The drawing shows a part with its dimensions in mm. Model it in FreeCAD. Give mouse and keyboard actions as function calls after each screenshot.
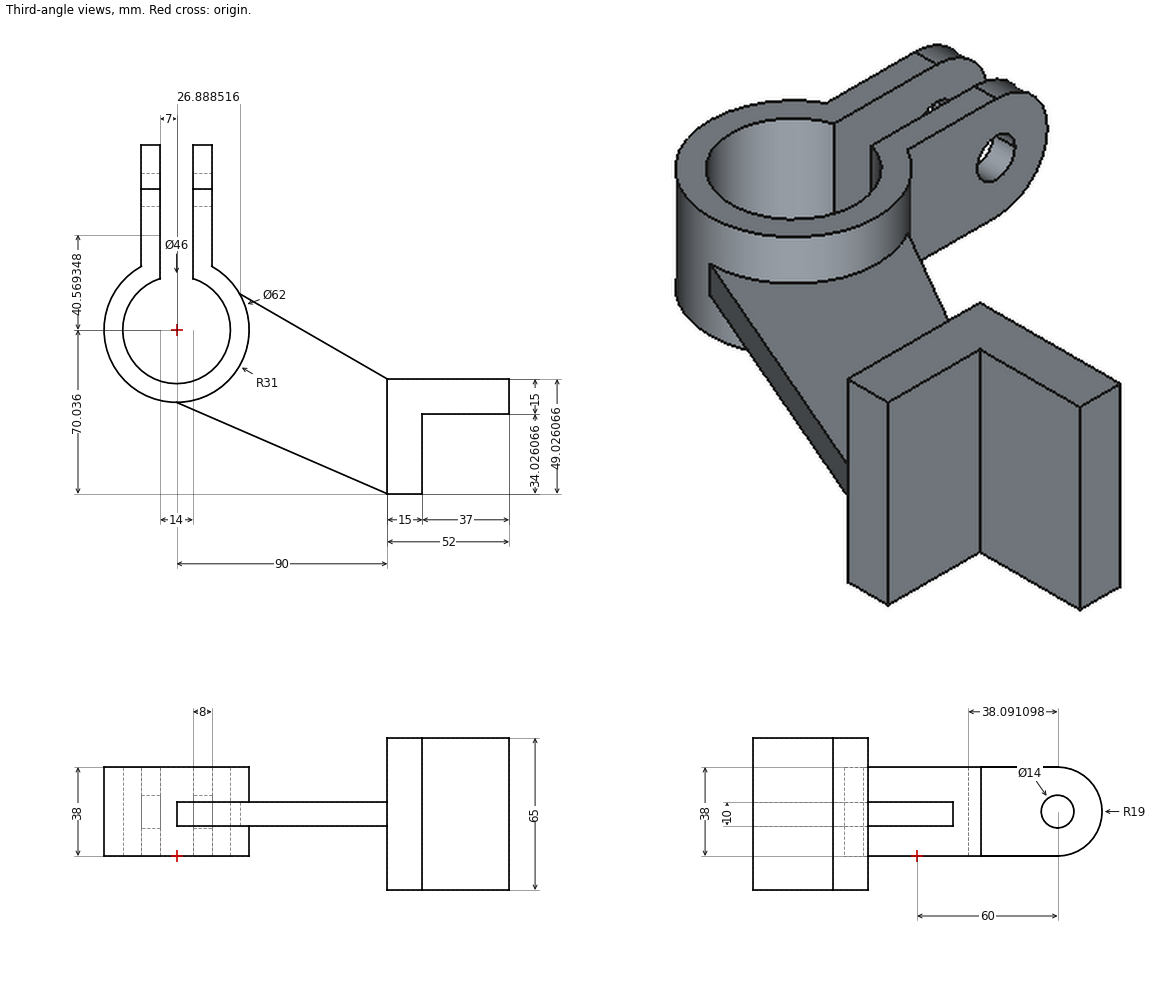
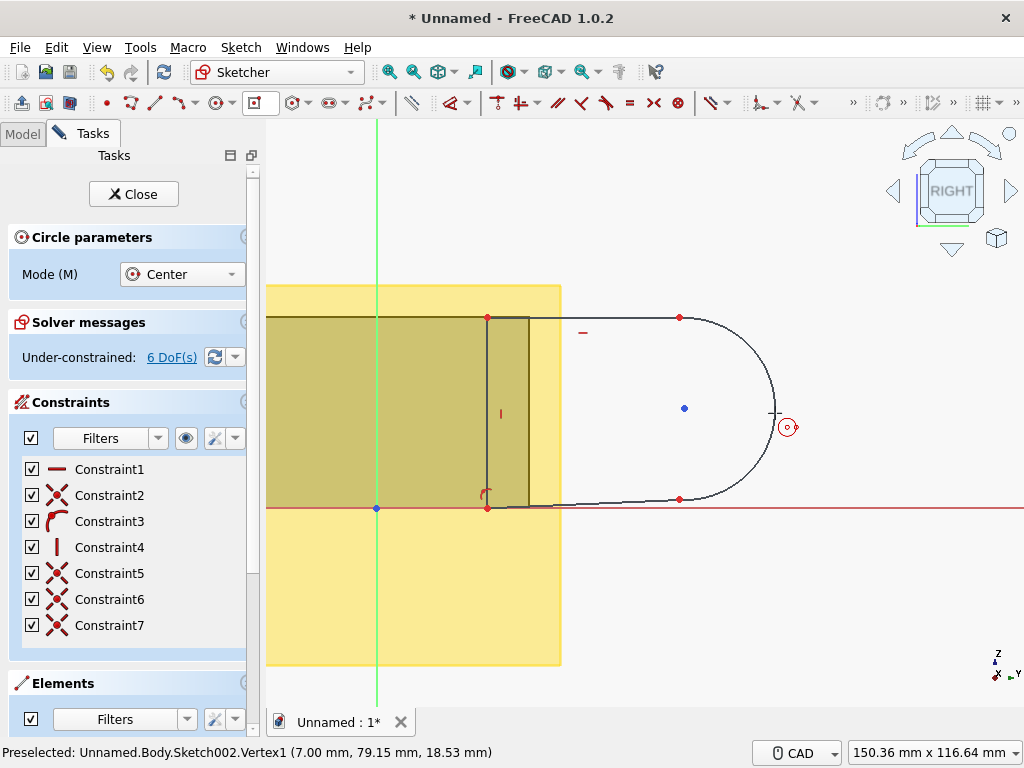
click(679, 413)
move(704, 388)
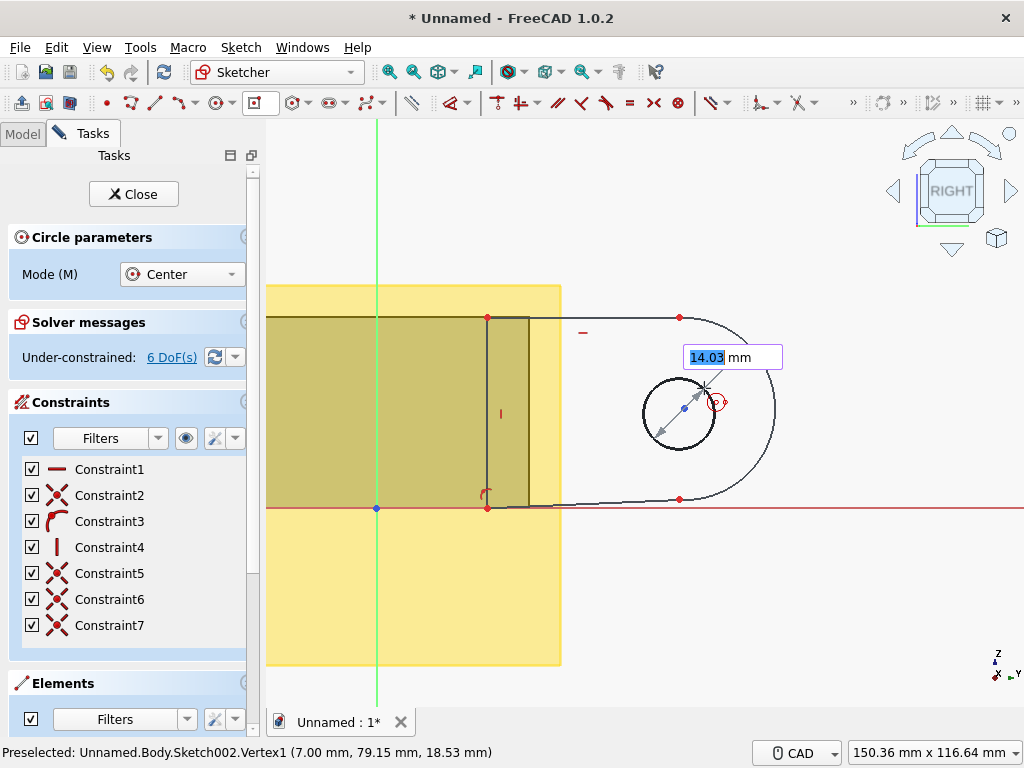
text(14)
key(Return)
key(Escape)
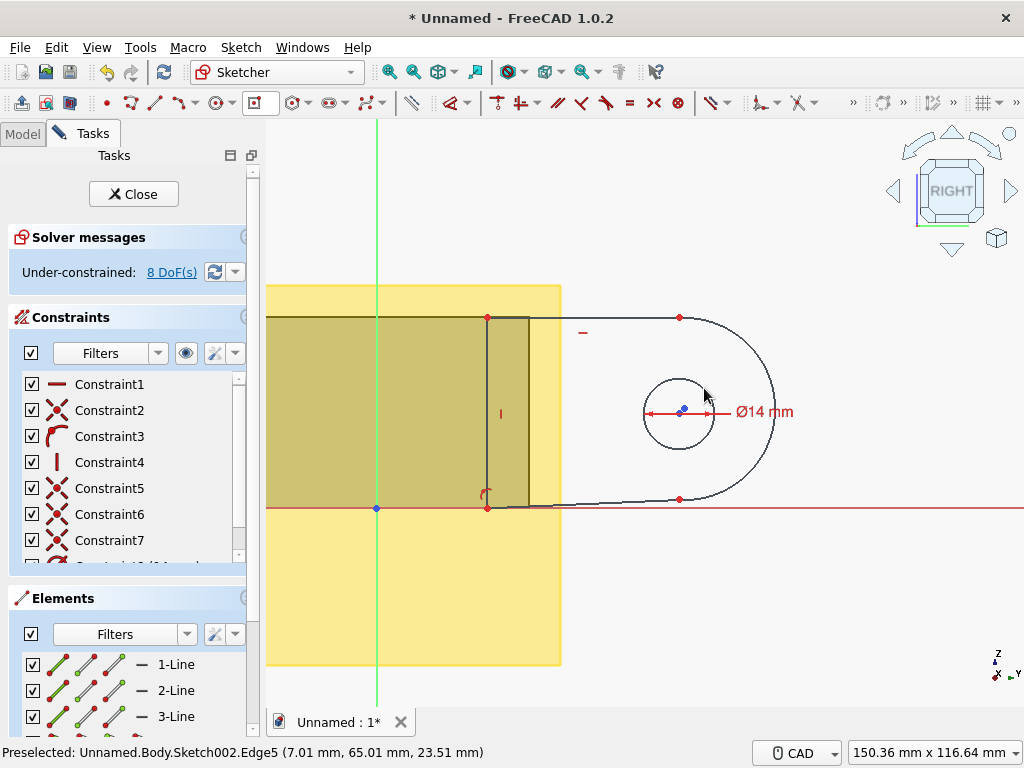
click(621, 318)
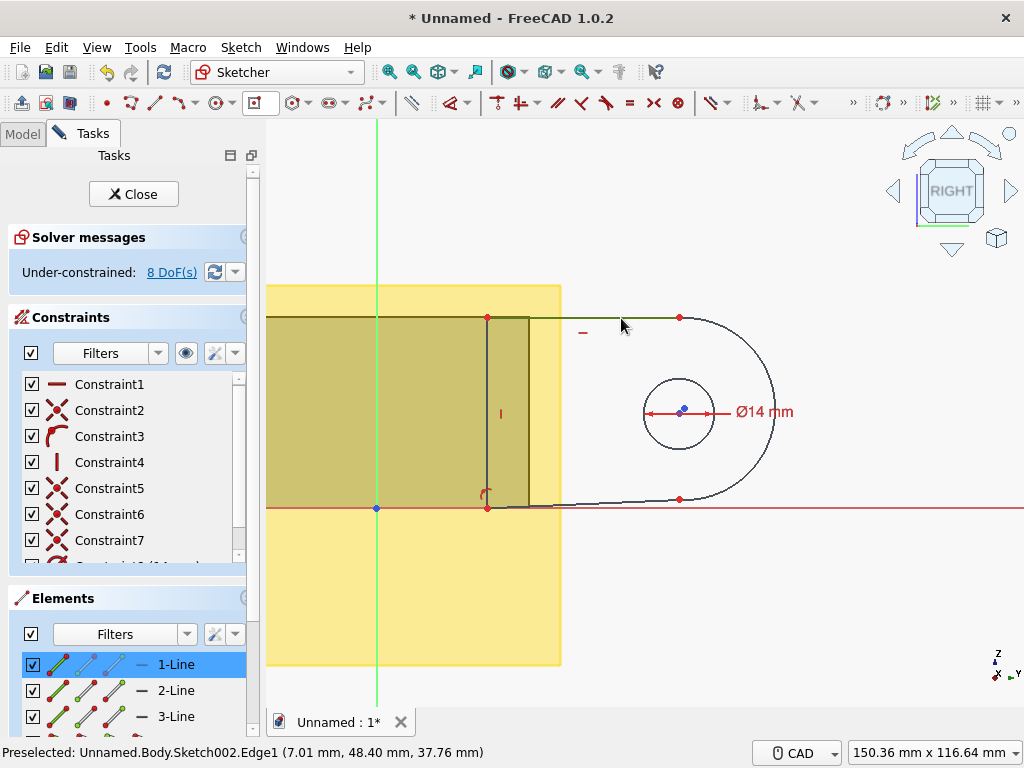
click(757, 464)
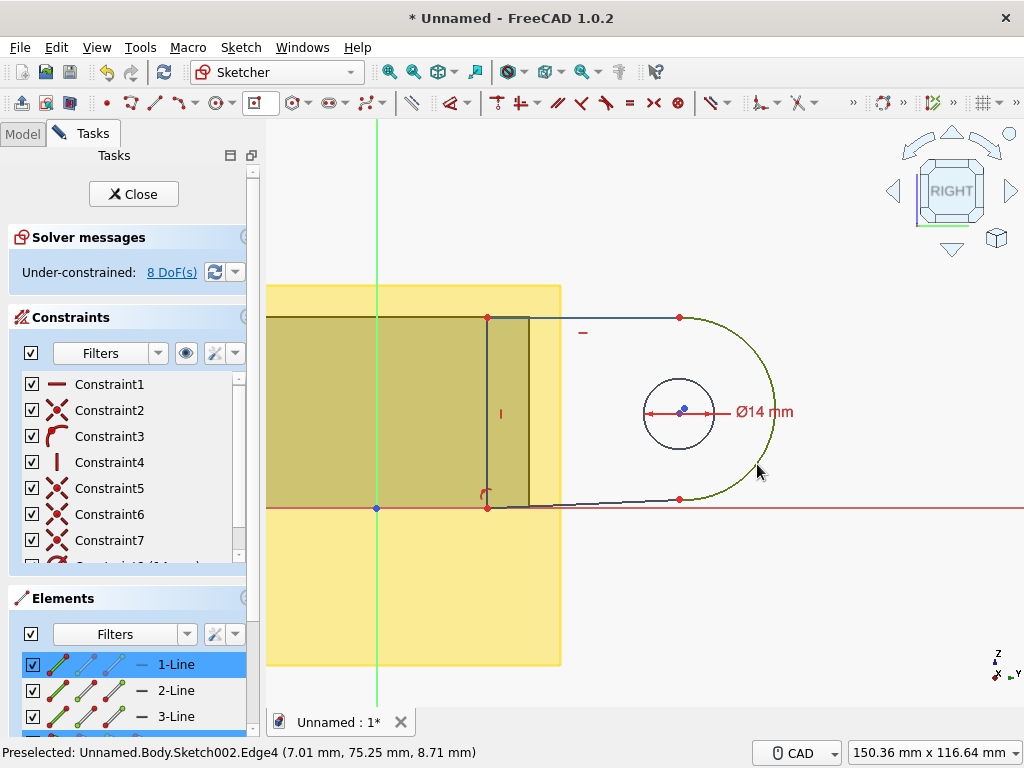
click(606, 104)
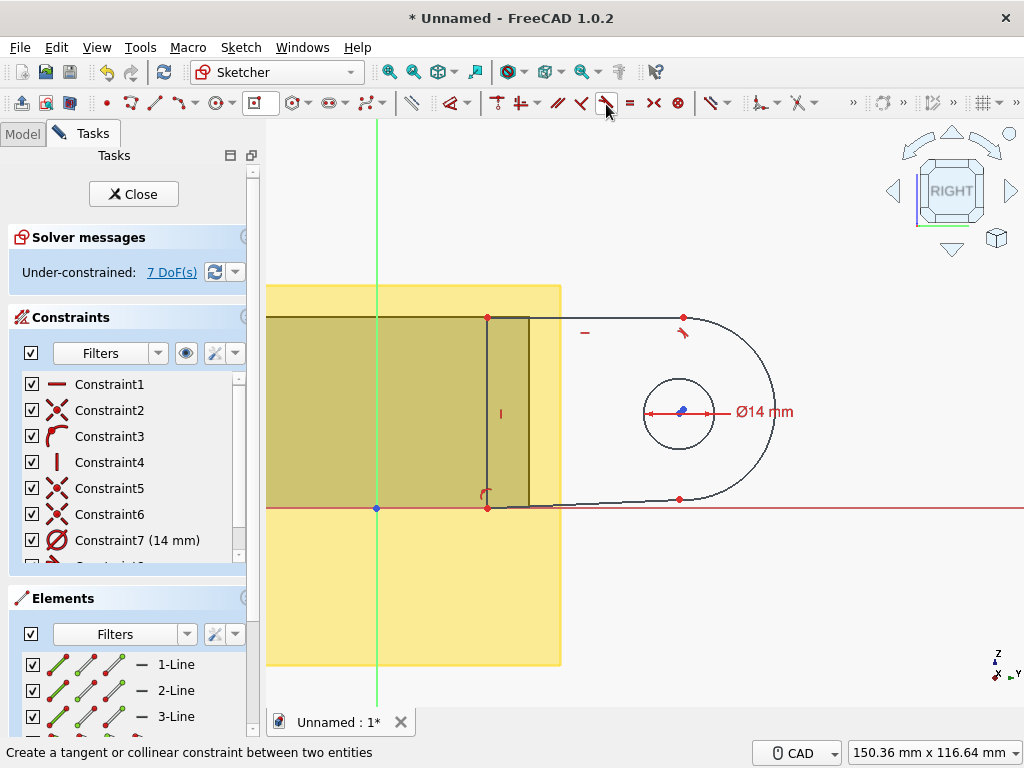
click(545, 506)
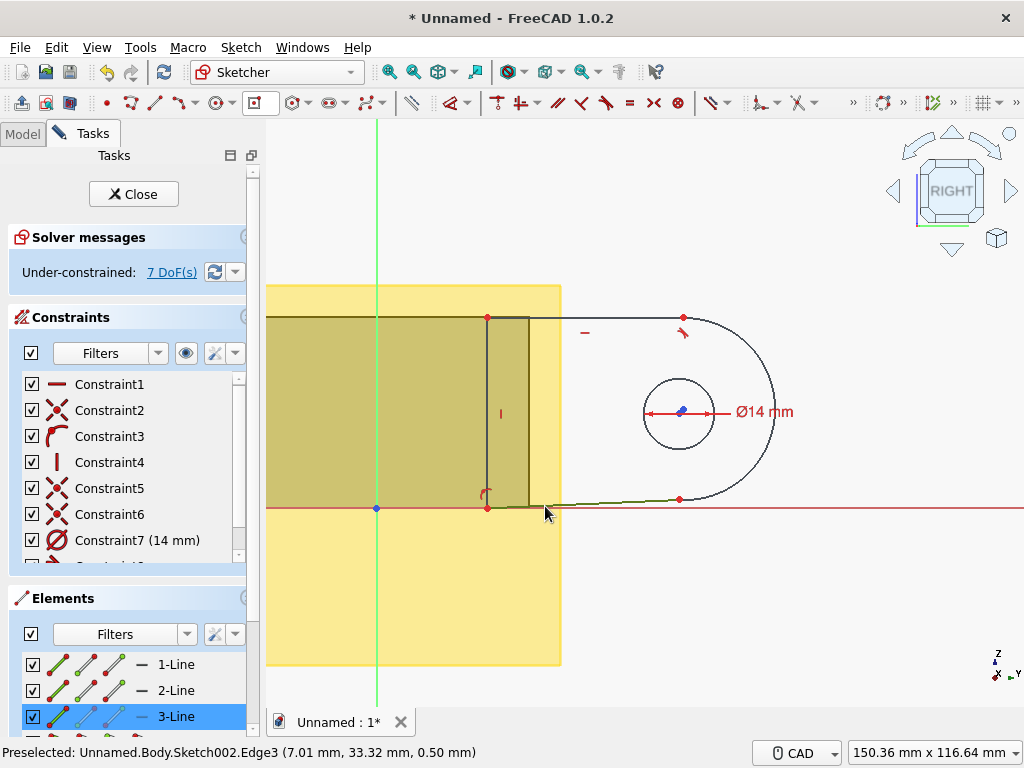
click(756, 465)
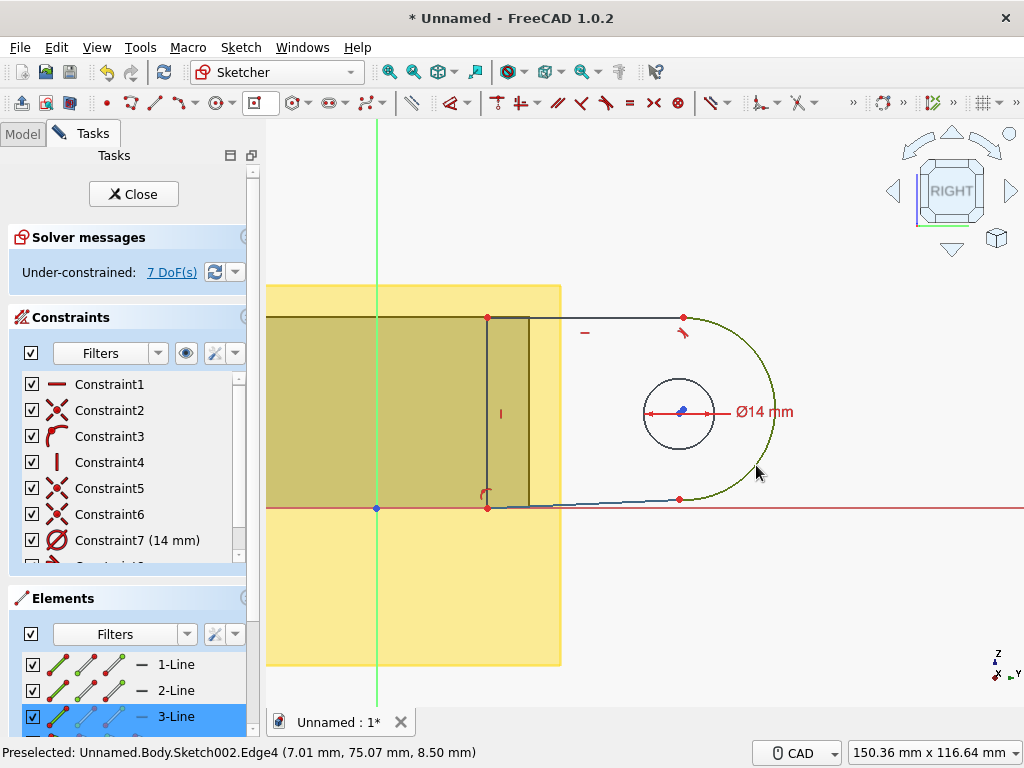
click(606, 104)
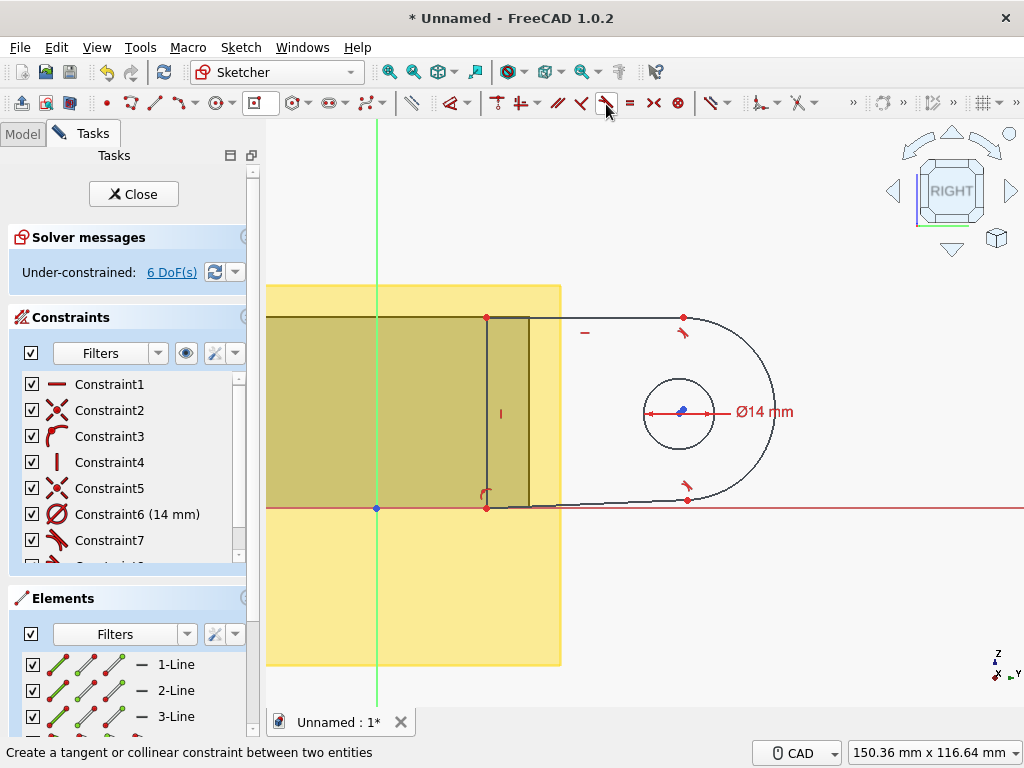
click(547, 506)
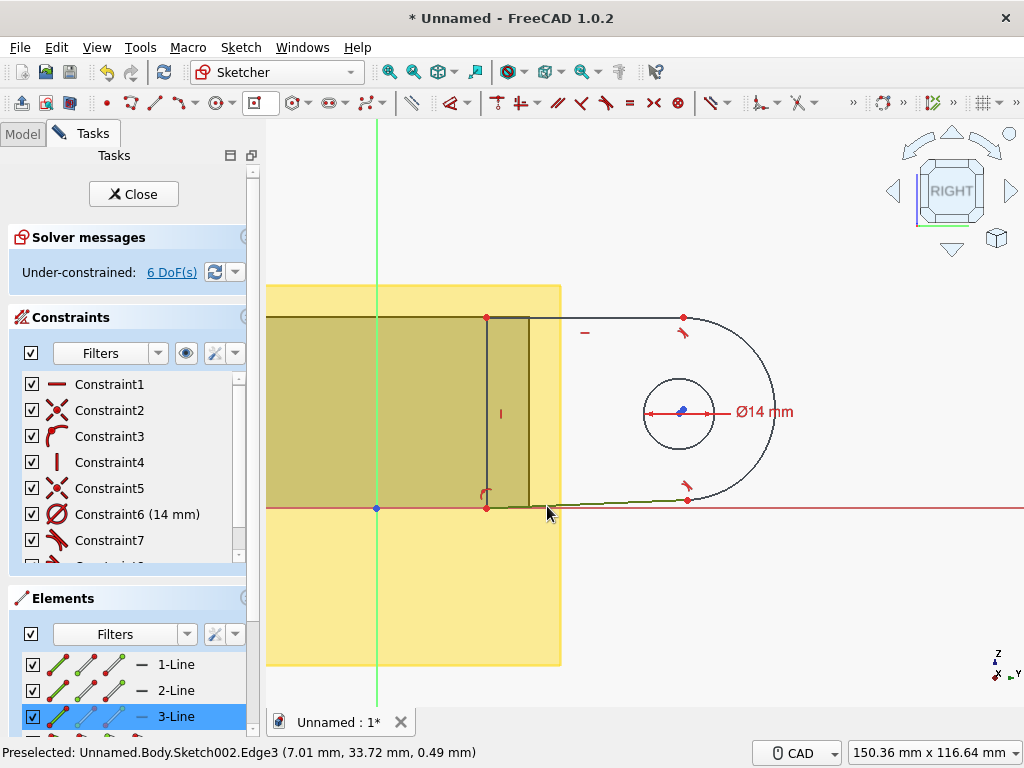
click(540, 104)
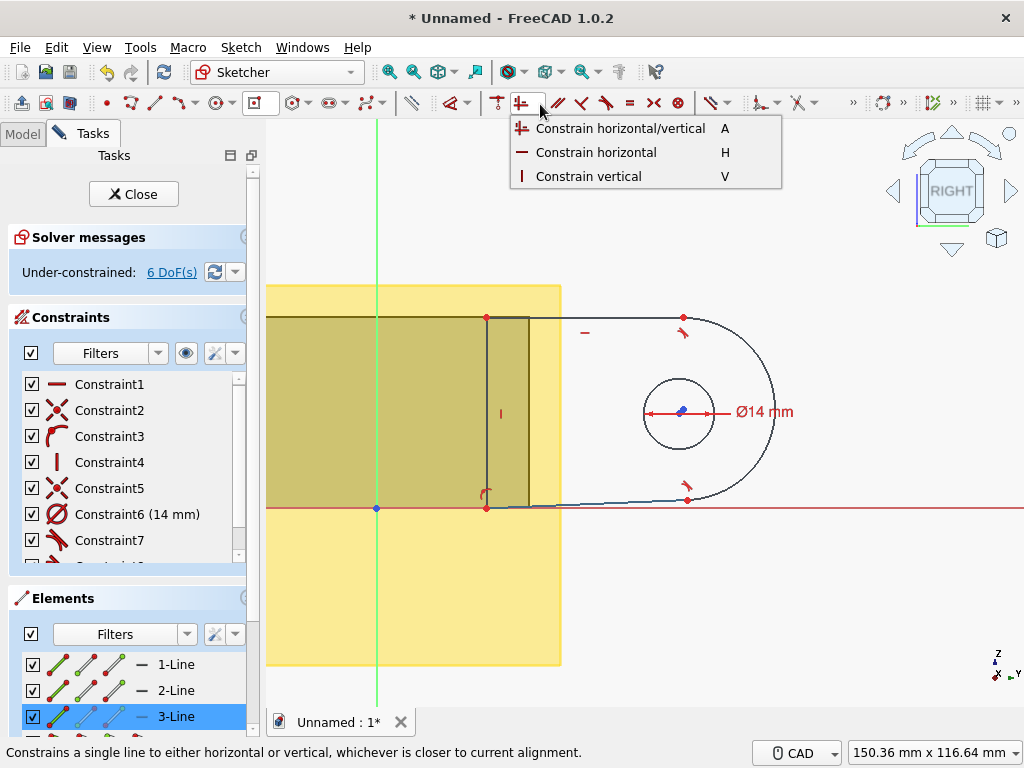
click(646, 152)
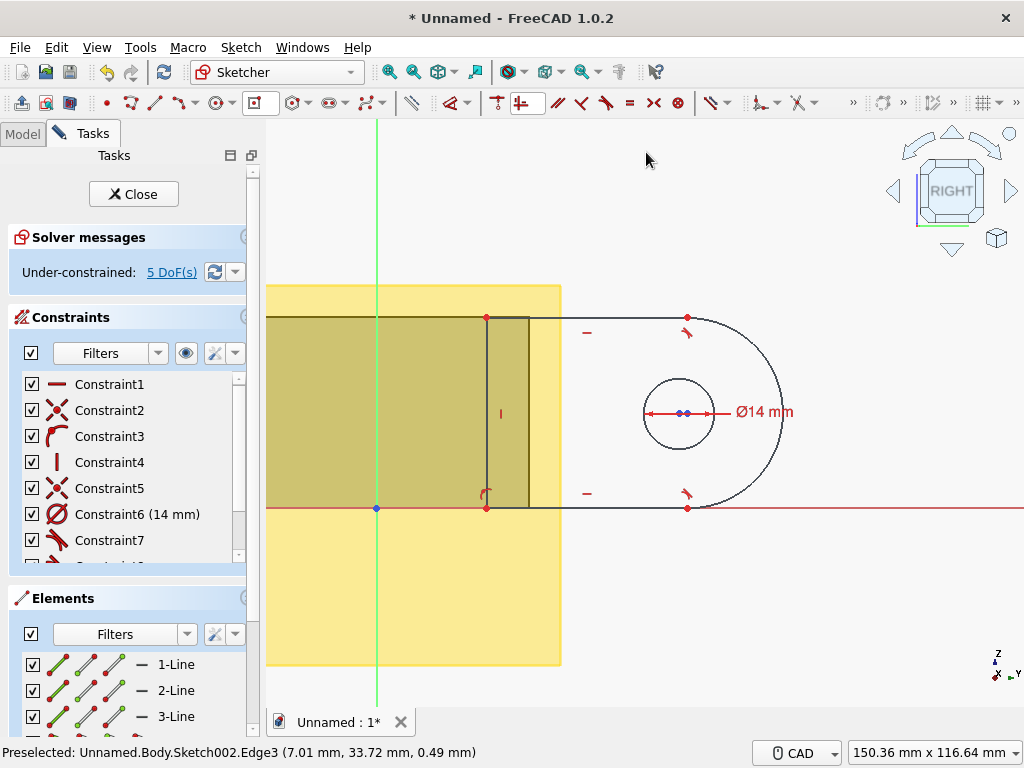
click(704, 389)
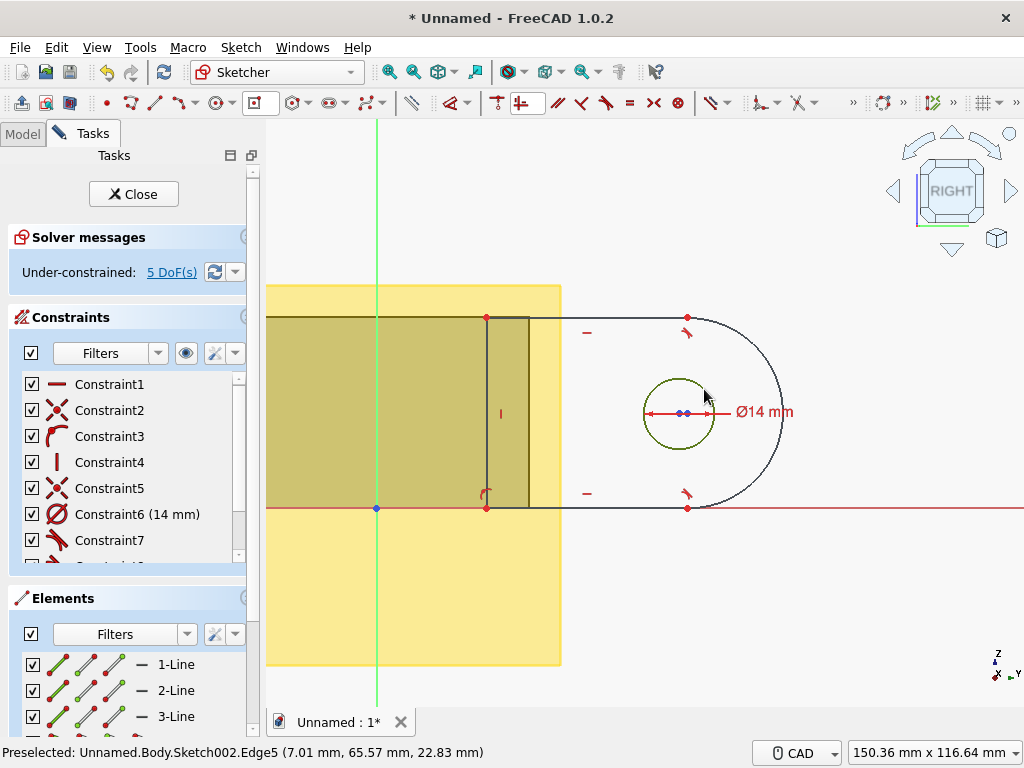
click(765, 469)